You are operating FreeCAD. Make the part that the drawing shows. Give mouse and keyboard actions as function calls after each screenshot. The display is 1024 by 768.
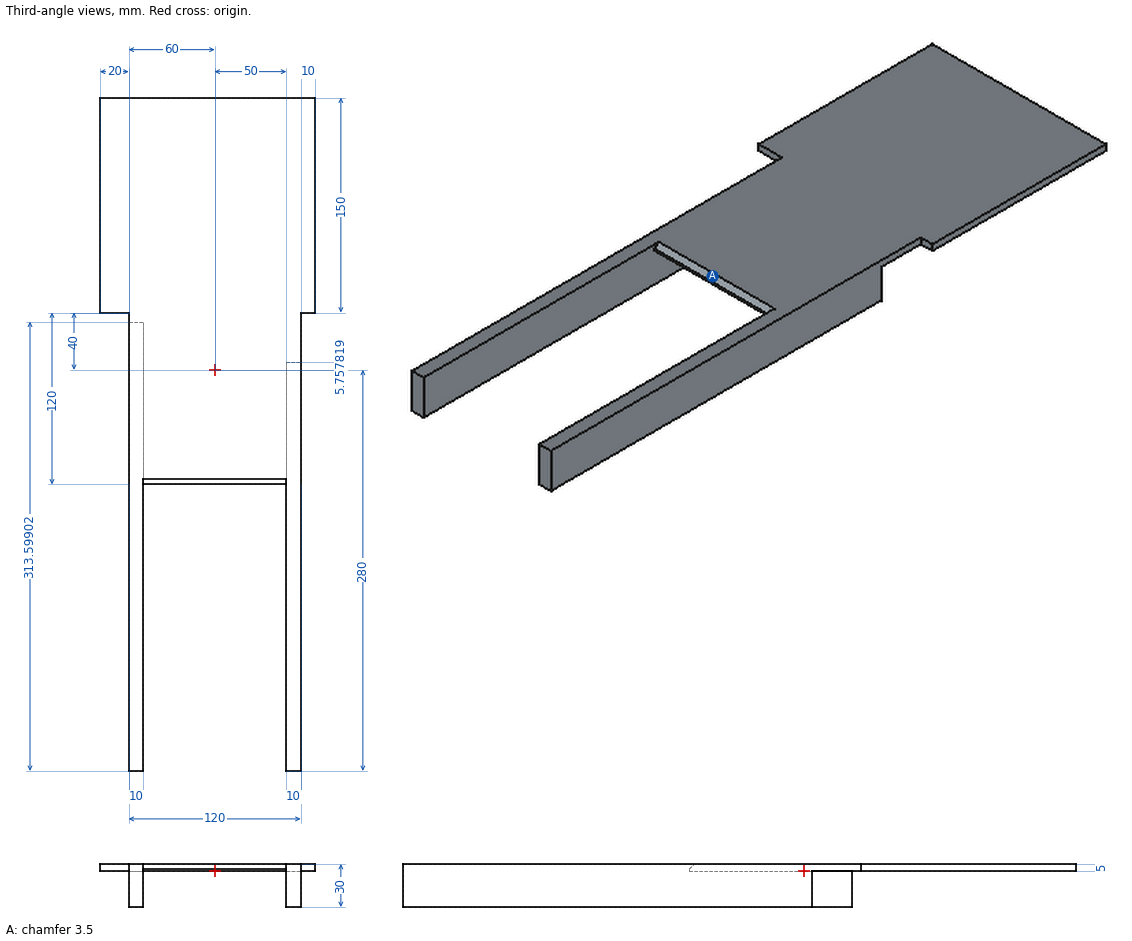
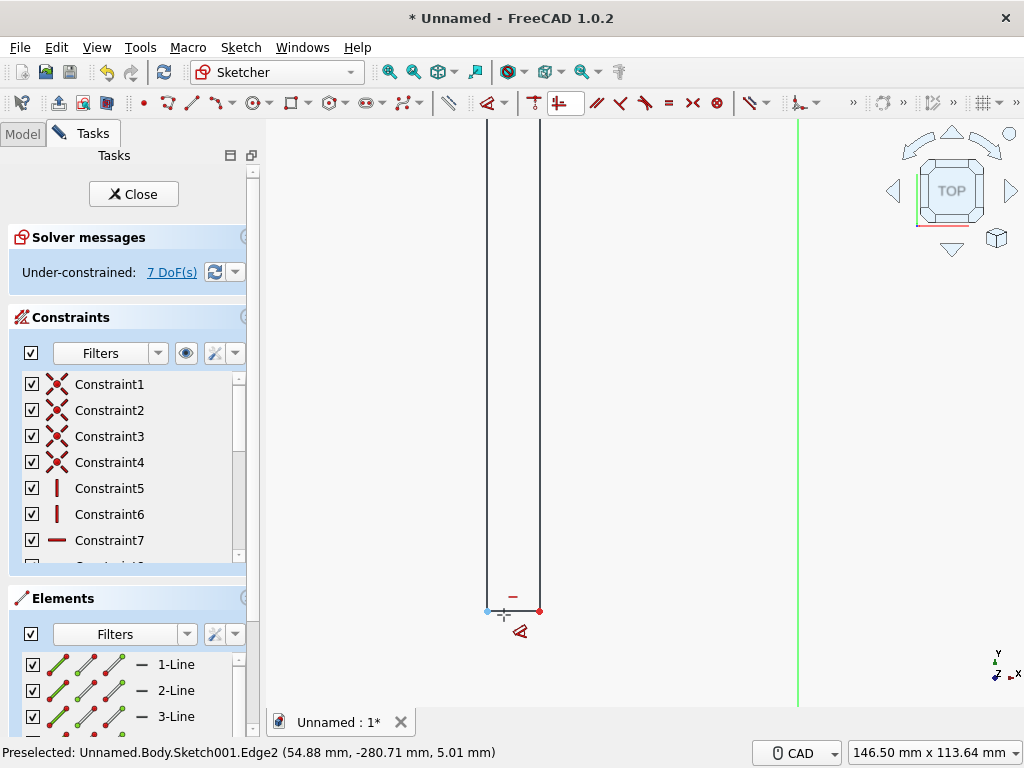
click(503, 611)
click(513, 645)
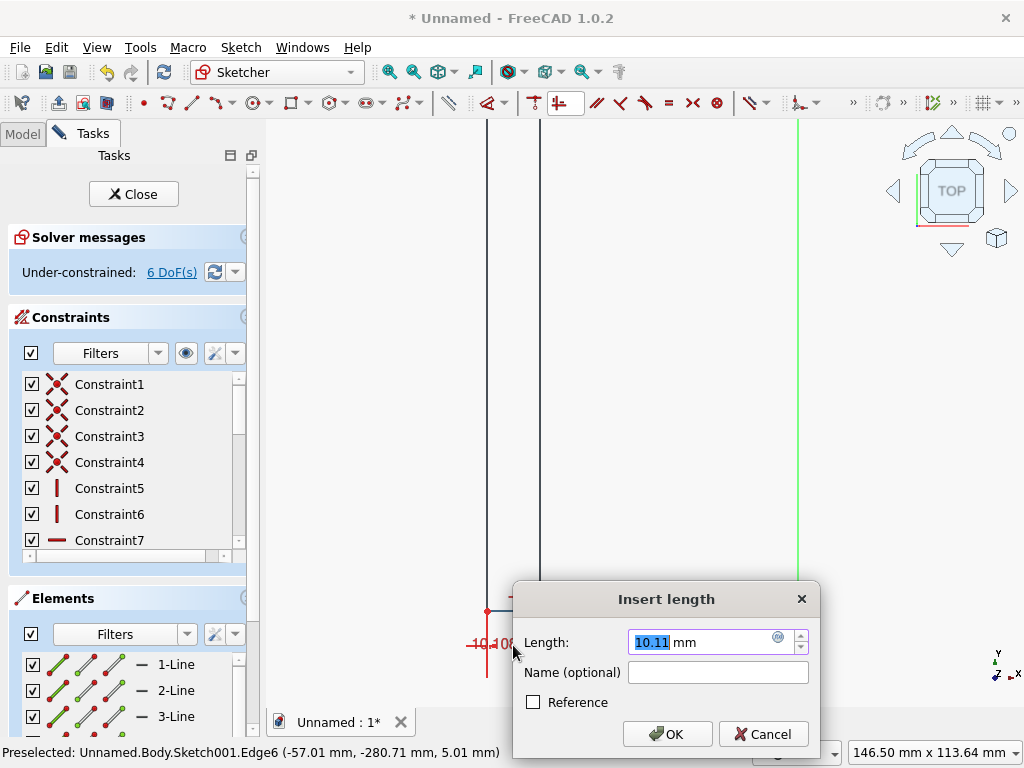
text(10)
key(Return)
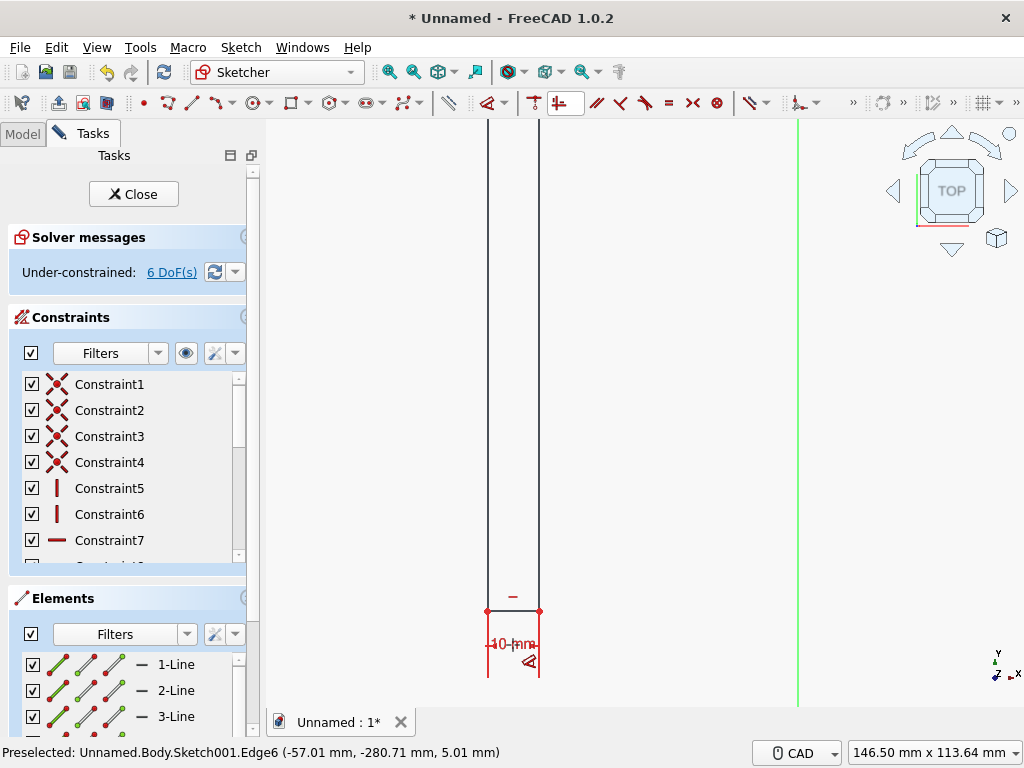
scroll(504, 615, down, 7)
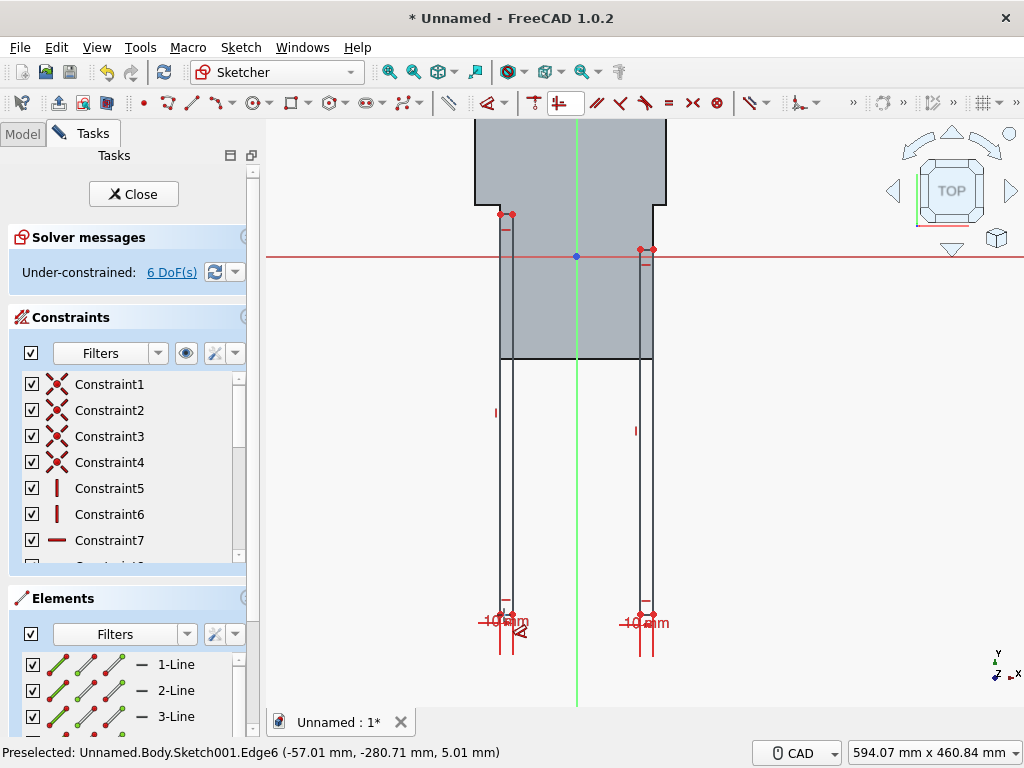
click(640, 250)
click(609, 216)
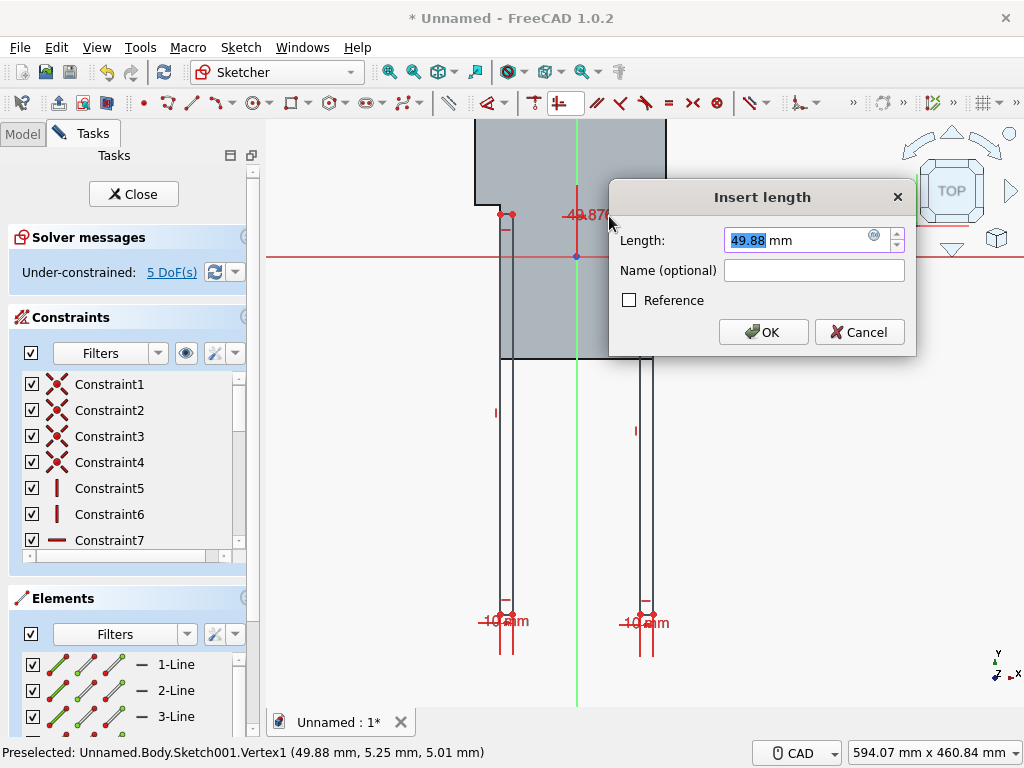
text(50)
key(Return)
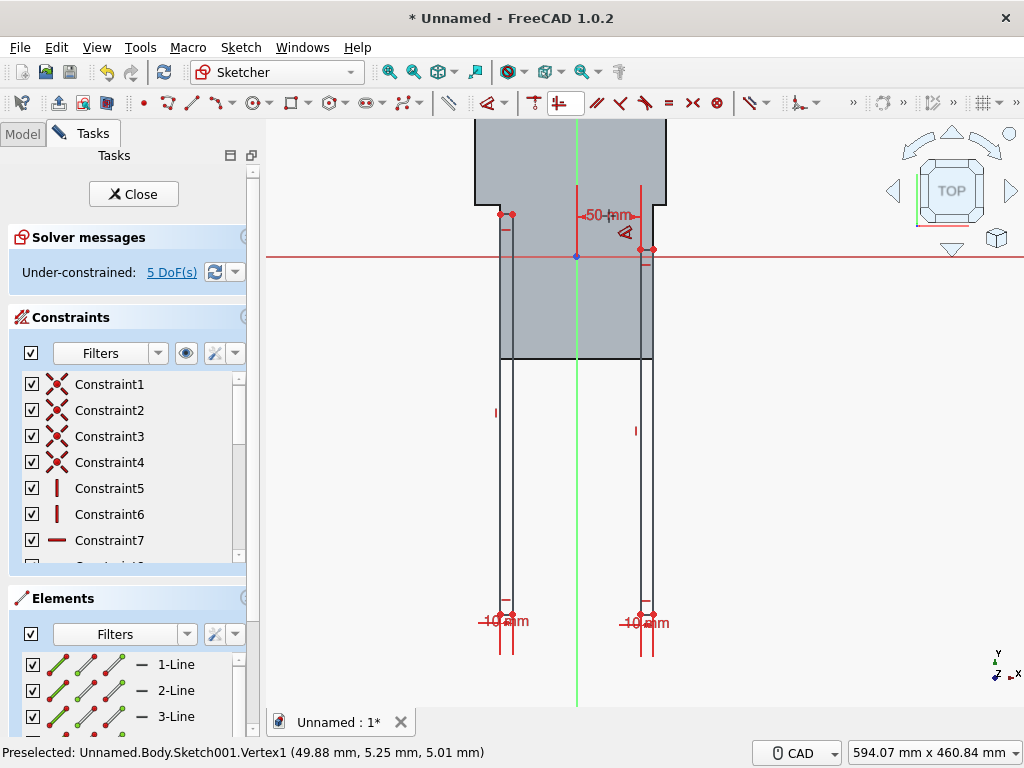
click(500, 214)
click(538, 180)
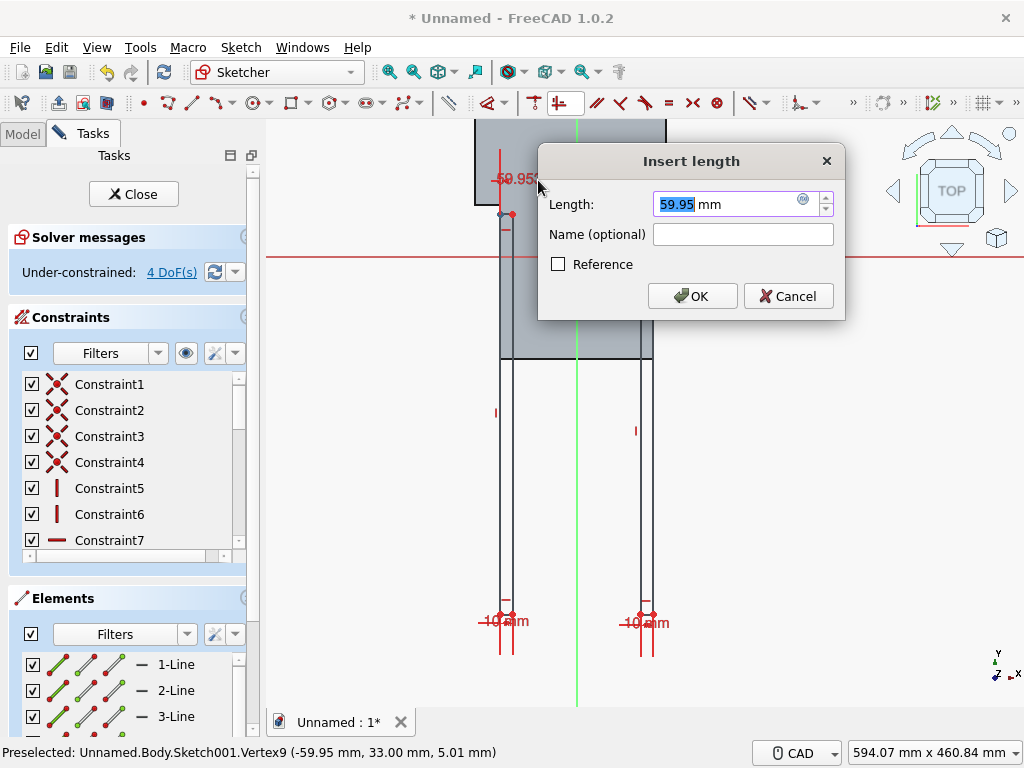
text(60)
key(Return)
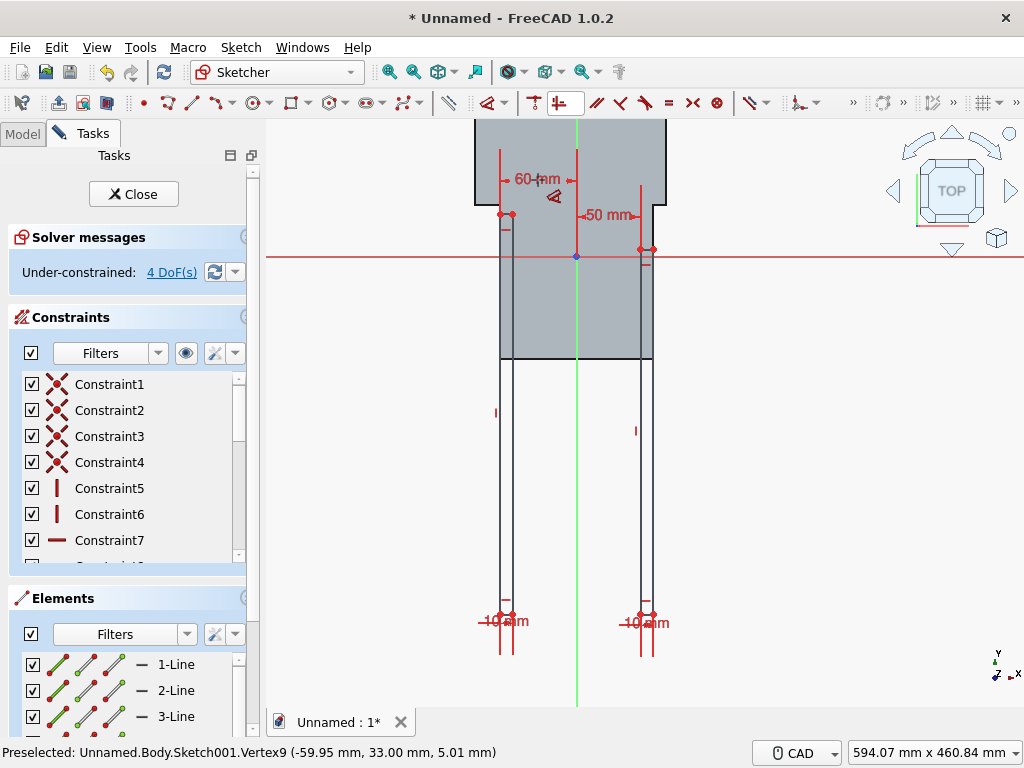
click(641, 615)
click(675, 436)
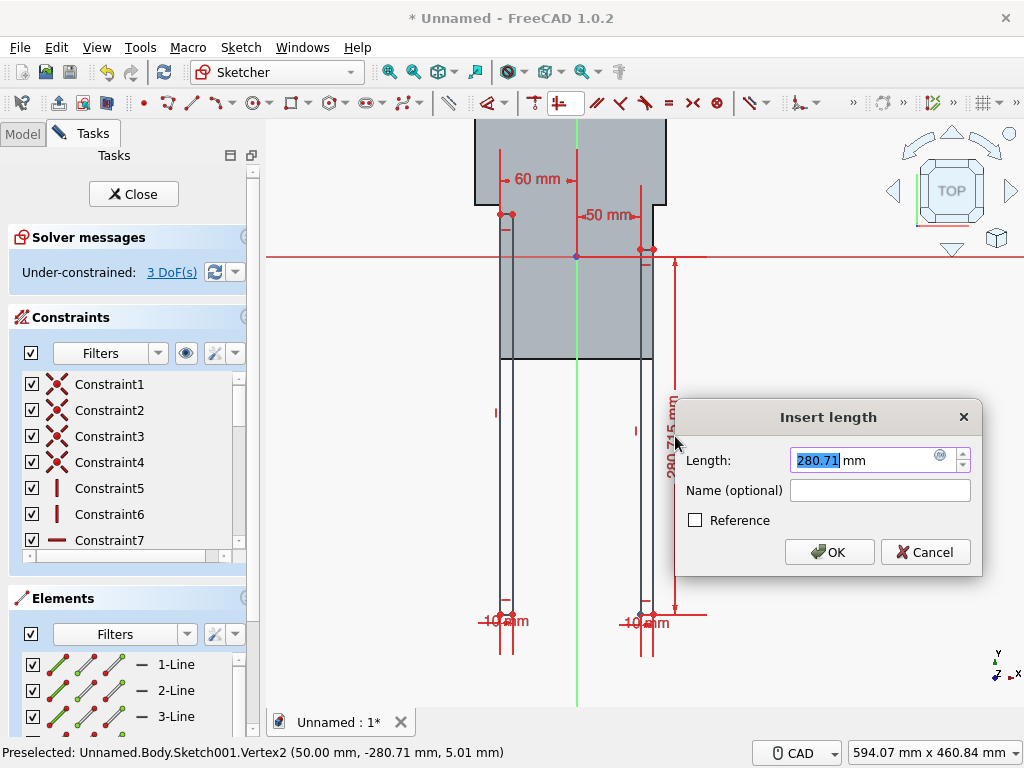
text(280)
key(Return)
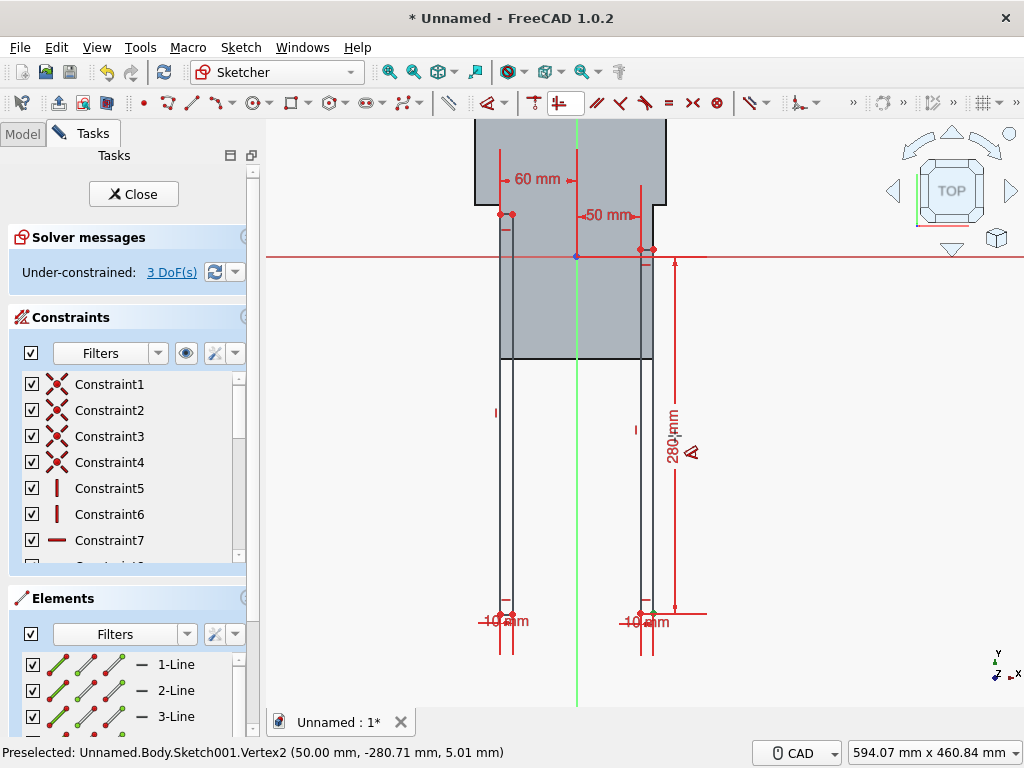
click(500, 615)
click(466, 436)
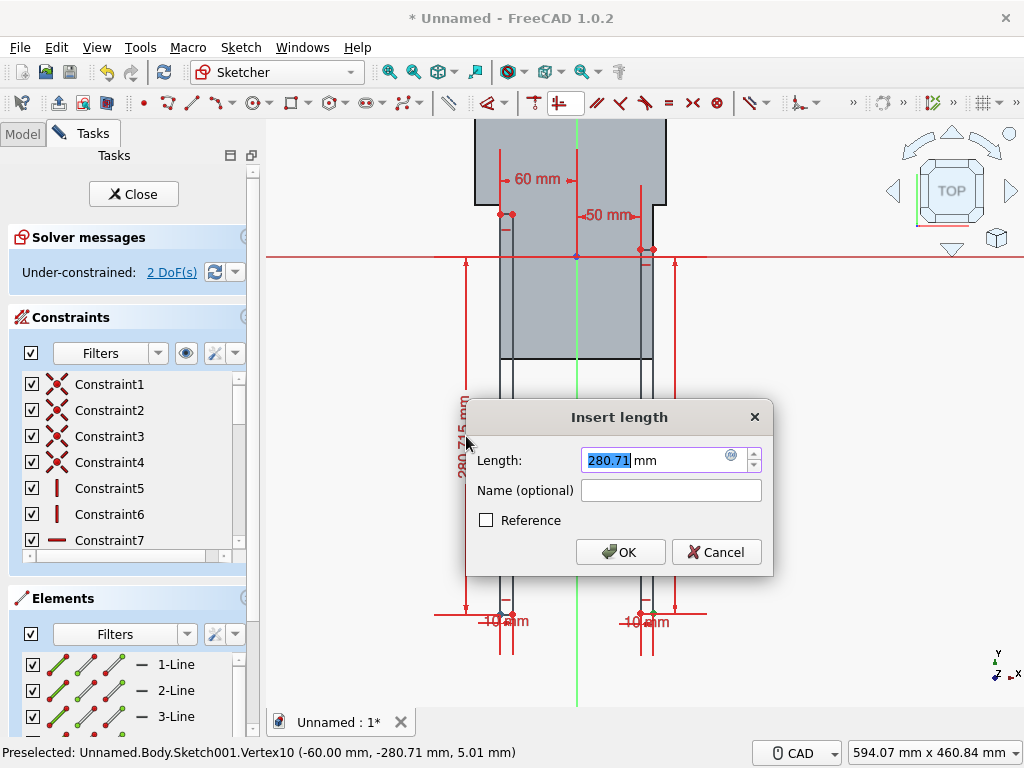
text(280)
key(Return)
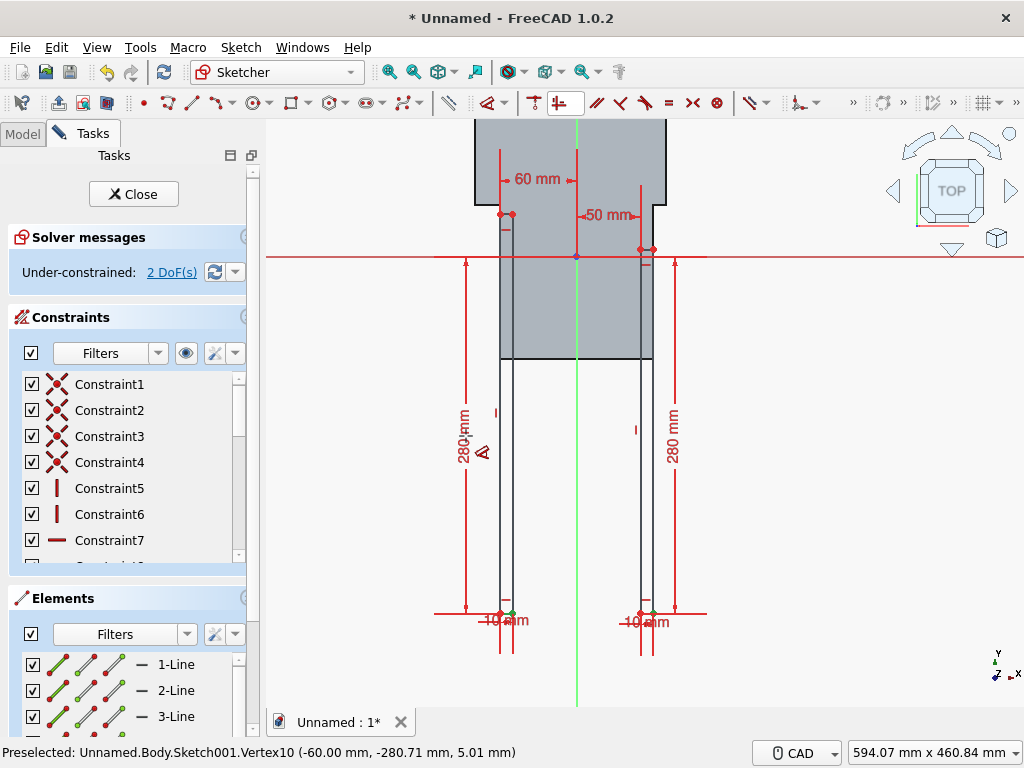
click(500, 334)
click(466, 414)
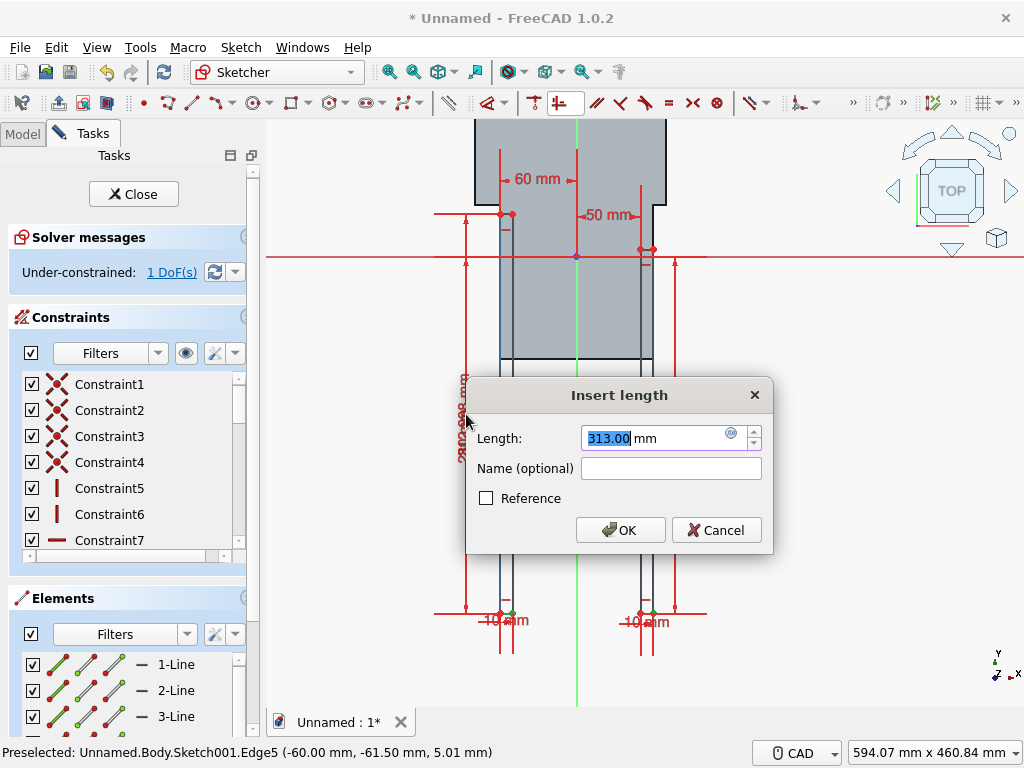
text(313.59902)
key(Return)